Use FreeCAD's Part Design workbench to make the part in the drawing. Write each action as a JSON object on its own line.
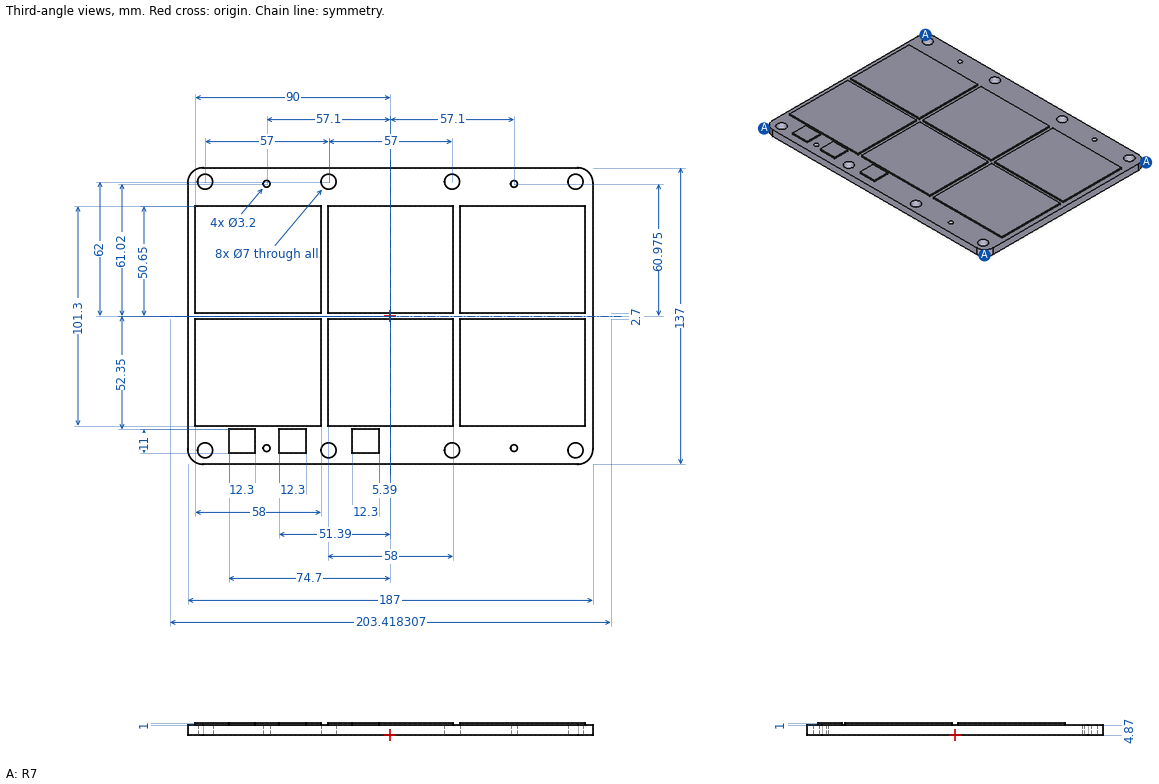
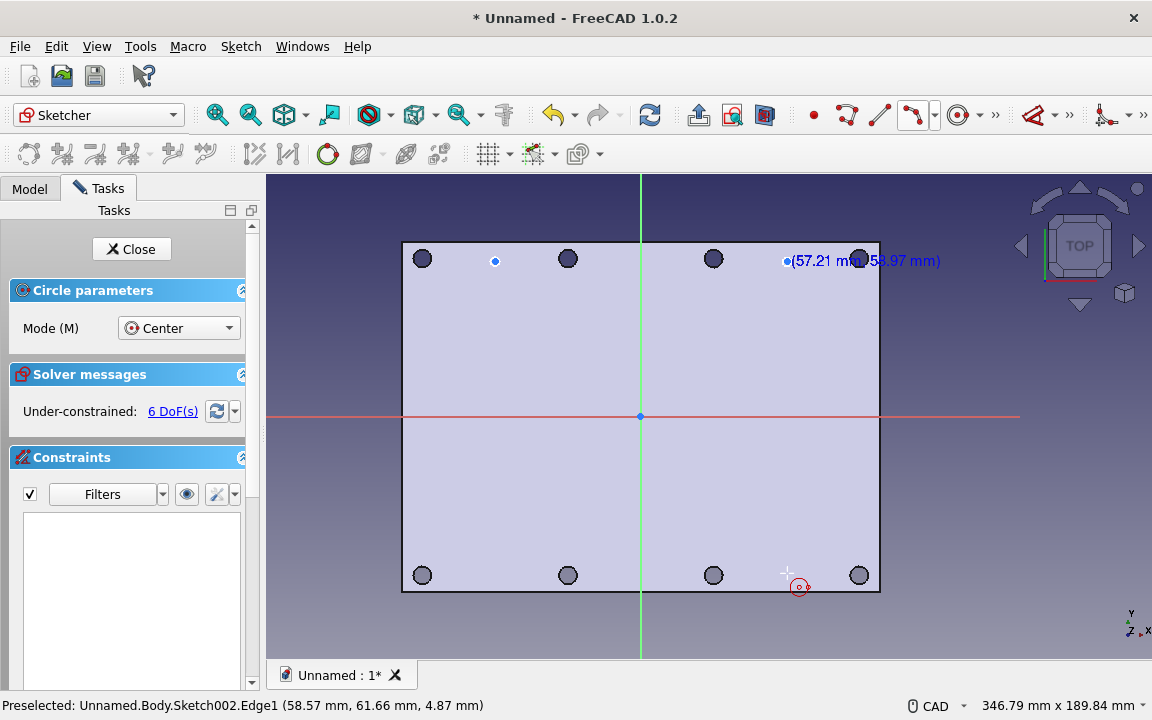
{"action": "left_click", "coordinate": [787, 573]}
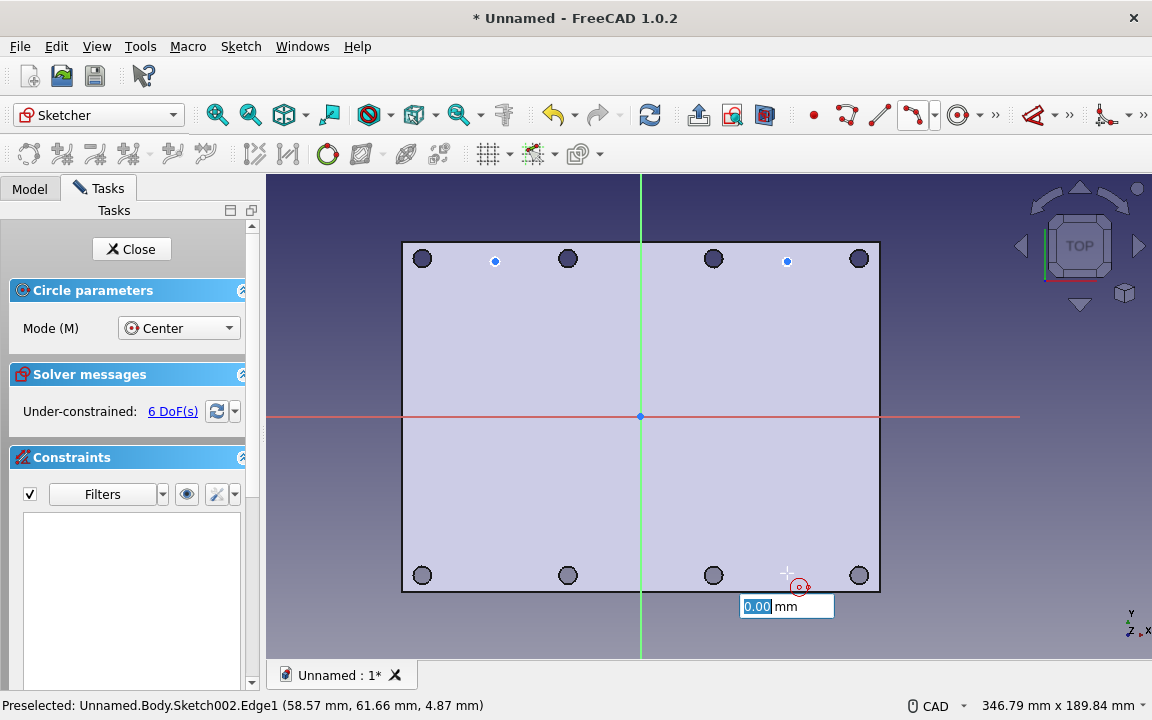
{"action": "scroll", "coordinate": [790, 570], "scroll_direction": "up", "scroll_amount": 7}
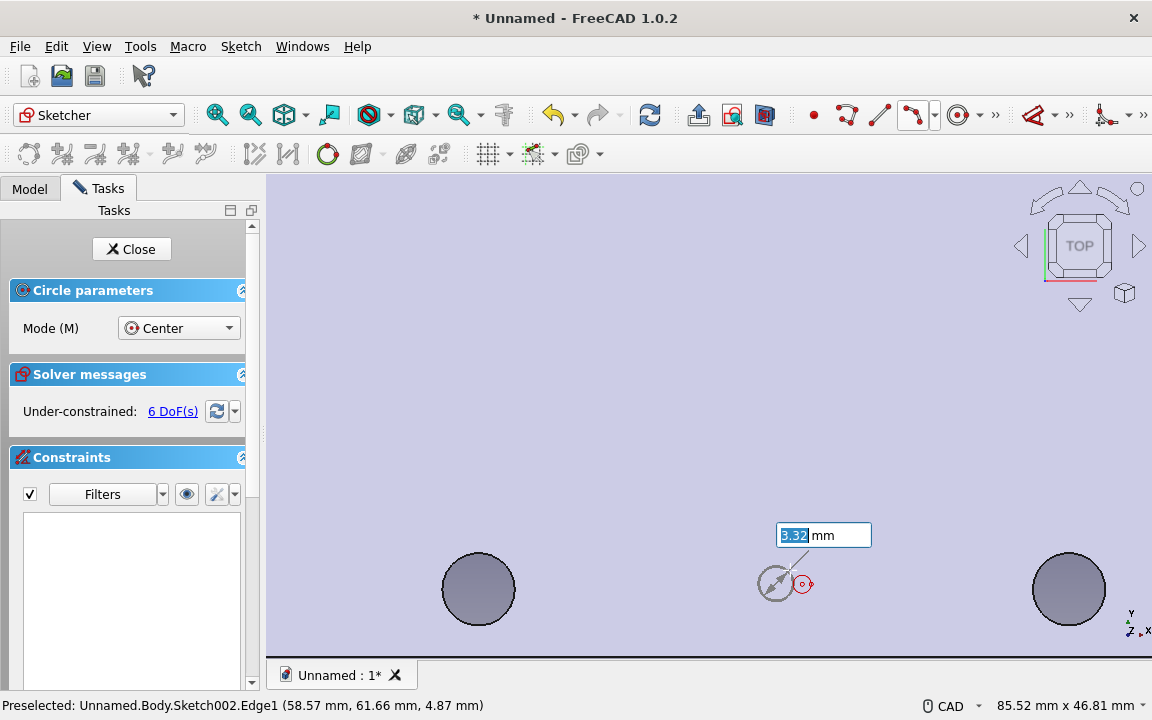
{"action": "left_click", "coordinate": [787, 567]}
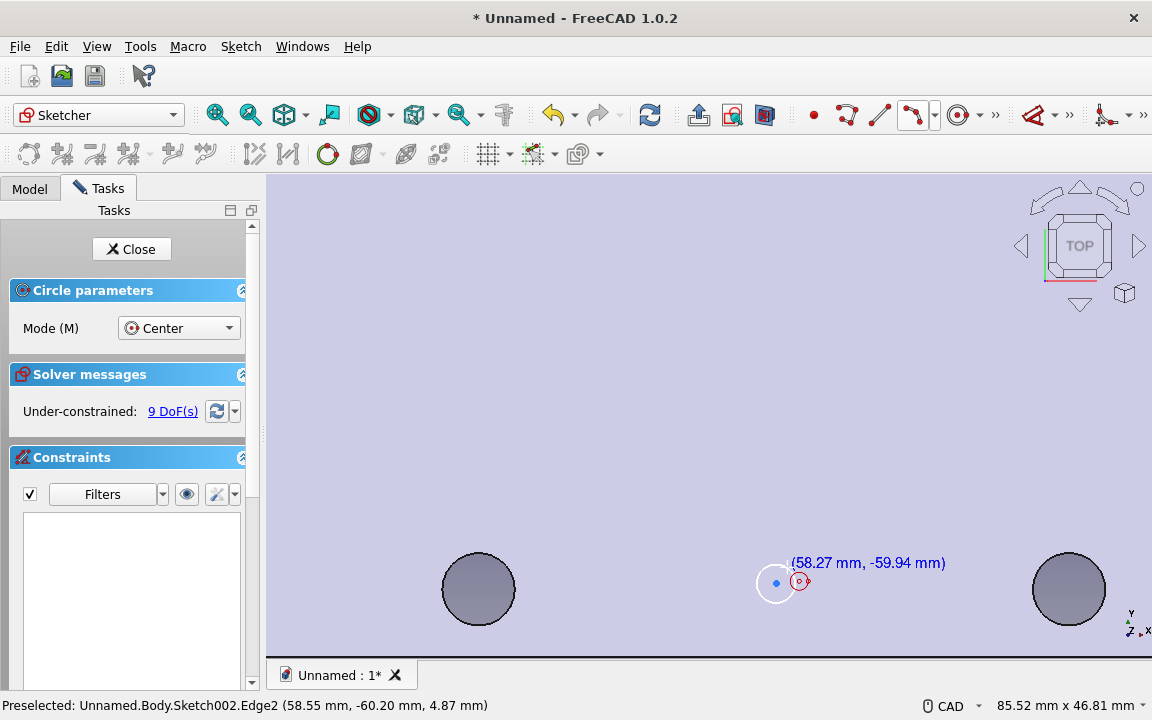
{"action": "scroll", "coordinate": [790, 570], "scroll_direction": "down", "scroll_amount": 7}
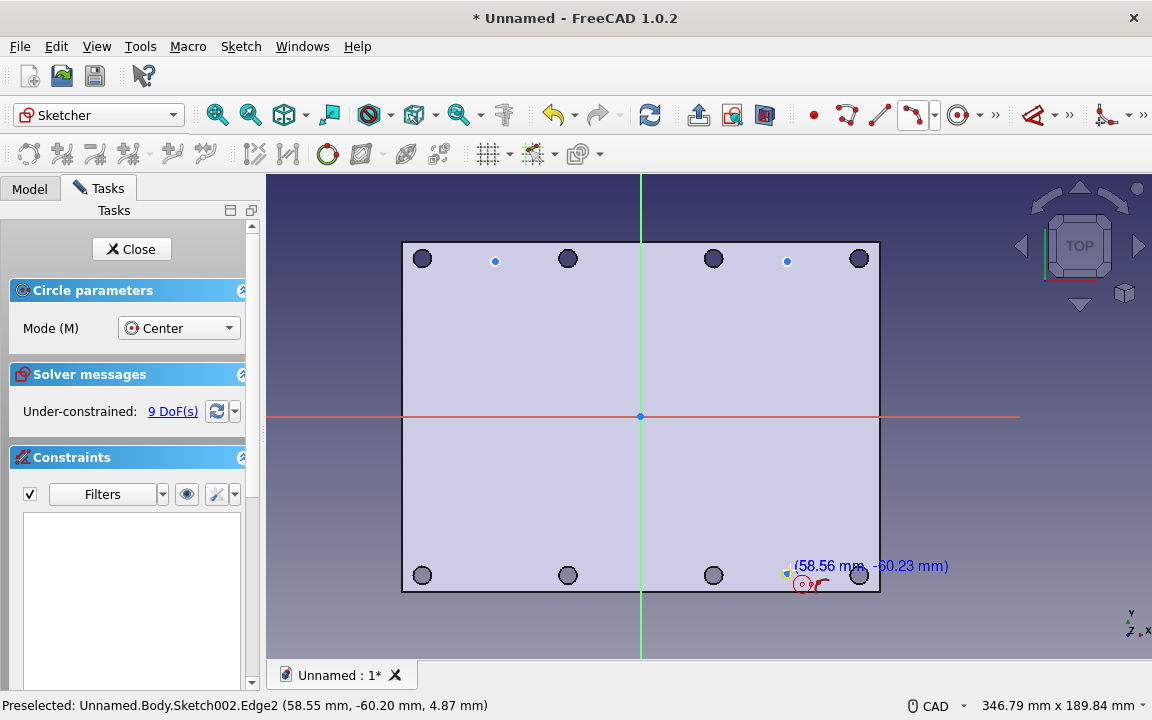
{"action": "scroll", "coordinate": [495, 573], "scroll_direction": "up", "scroll_amount": 9}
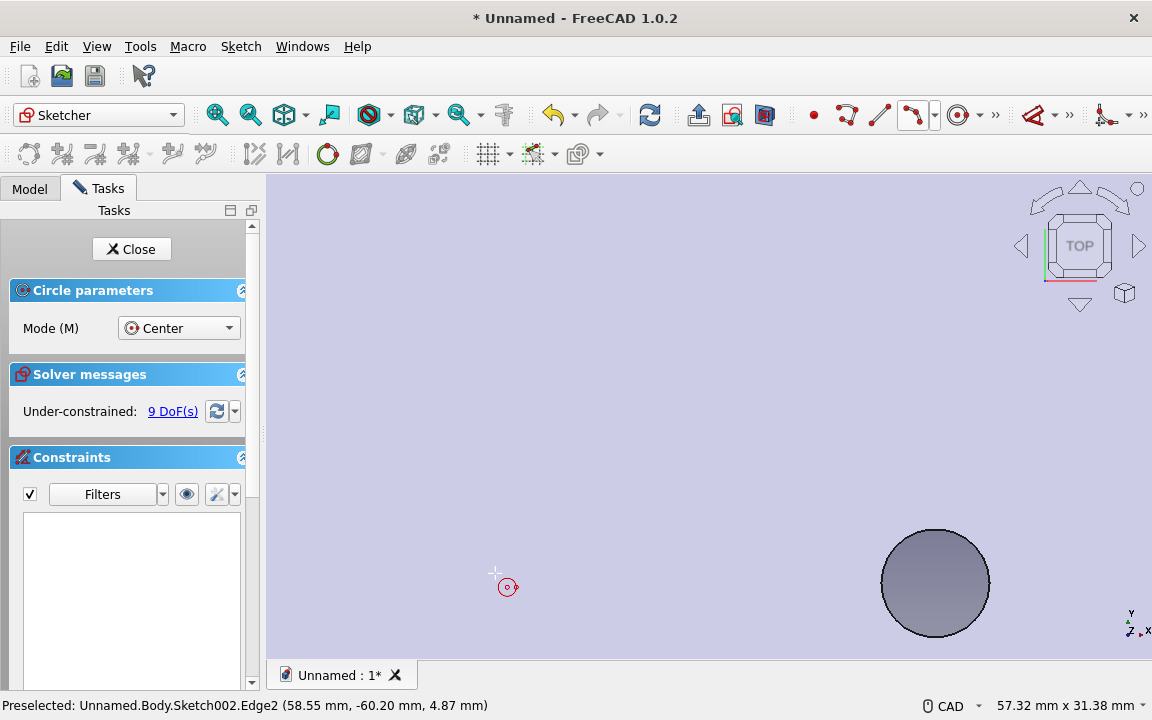
{"action": "scroll", "coordinate": [495, 573], "scroll_direction": "down", "scroll_amount": 9}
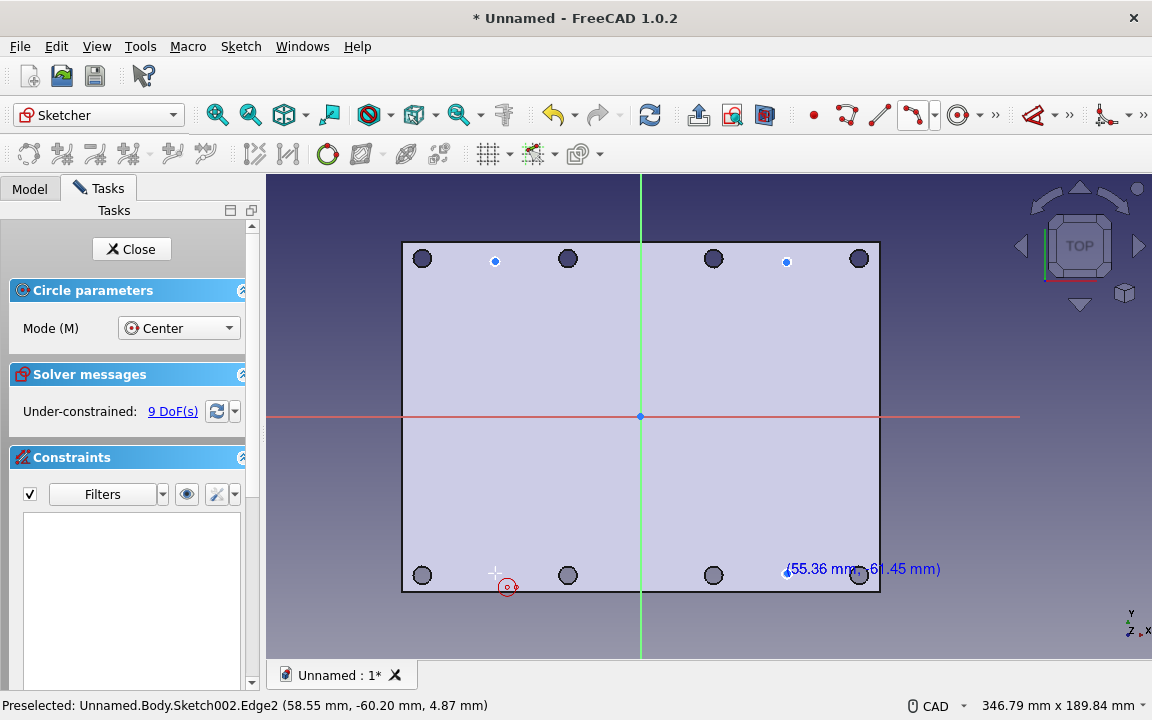
{"action": "left_click", "coordinate": [495, 573]}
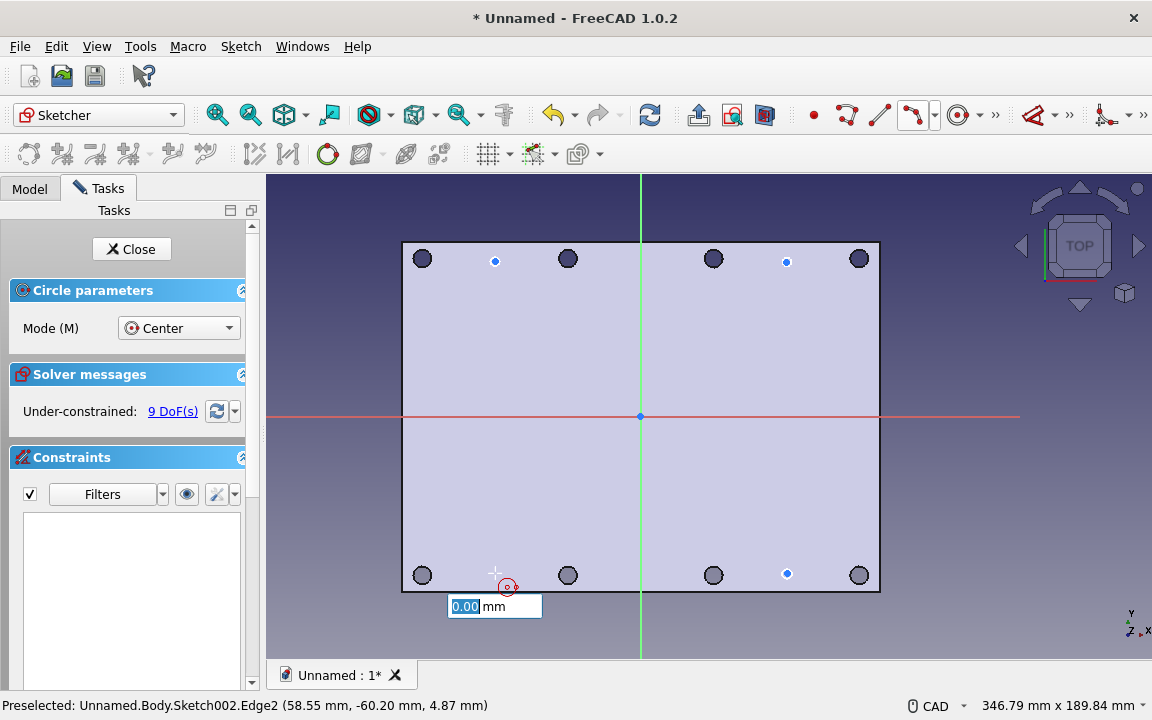
{"action": "scroll", "coordinate": [498, 570], "scroll_direction": "up", "scroll_amount": 7}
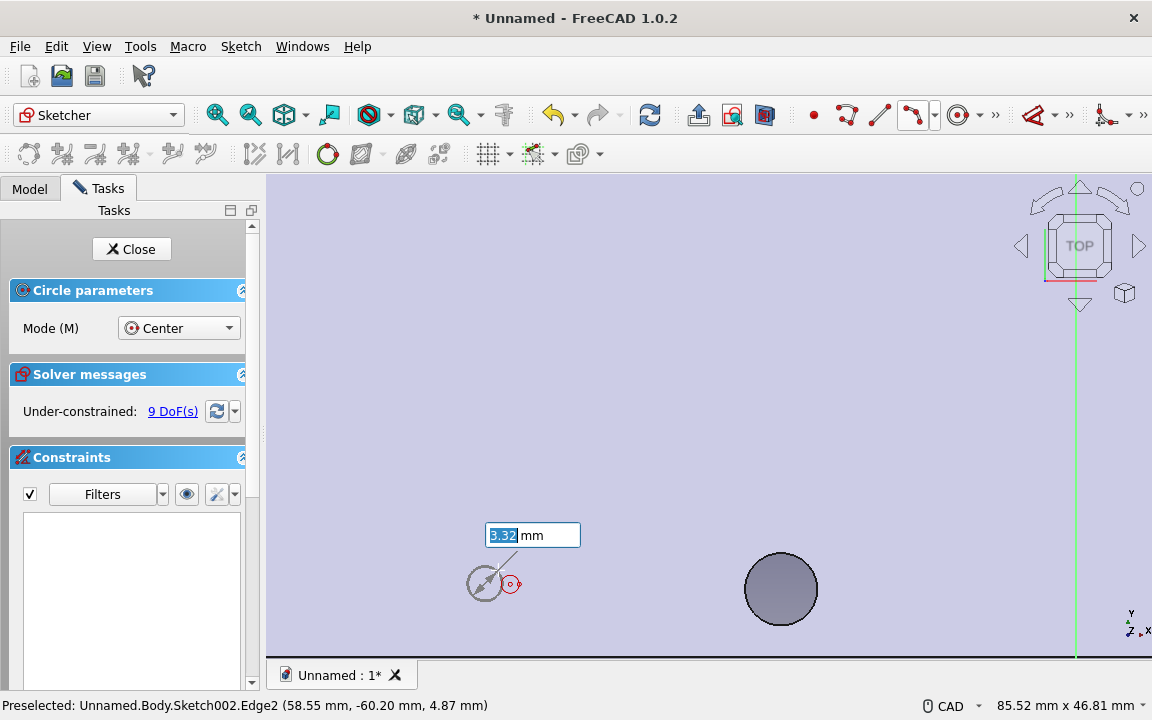
{"action": "left_click", "coordinate": [497, 567]}
{"action": "key", "text": "Escape"}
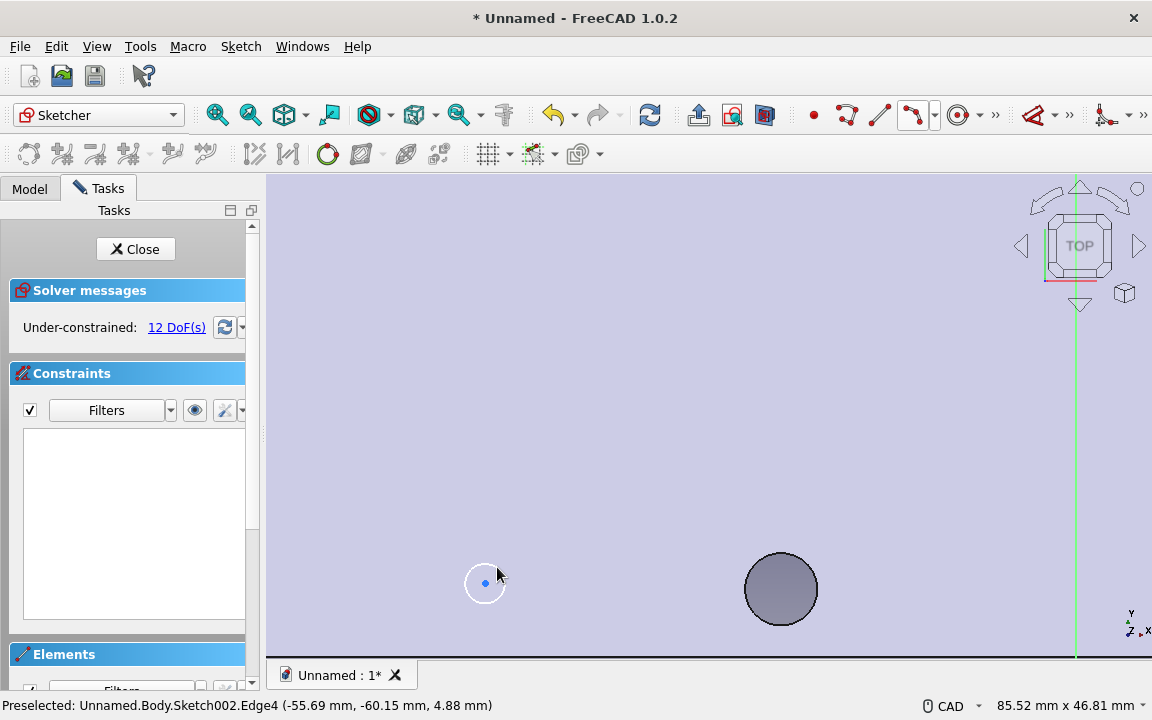
{"action": "scroll", "coordinate": [498, 570], "scroll_direction": "down", "scroll_amount": 7}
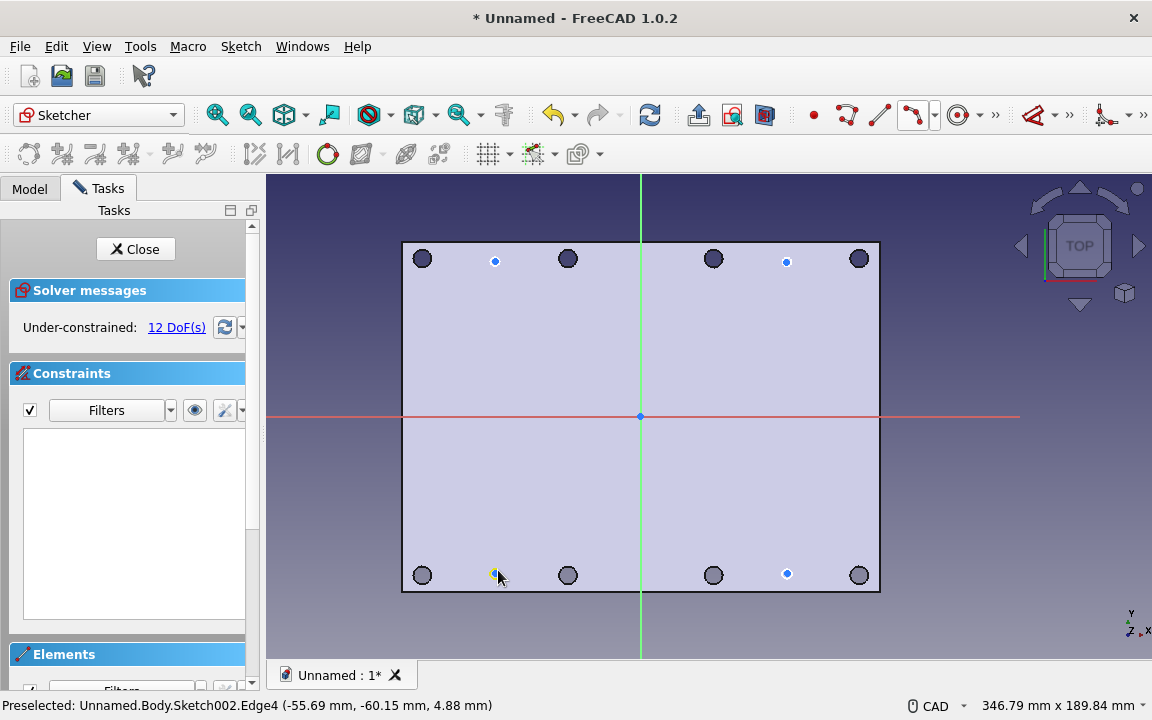
{"action": "scroll", "coordinate": [498, 259], "scroll_direction": "up", "scroll_amount": 6}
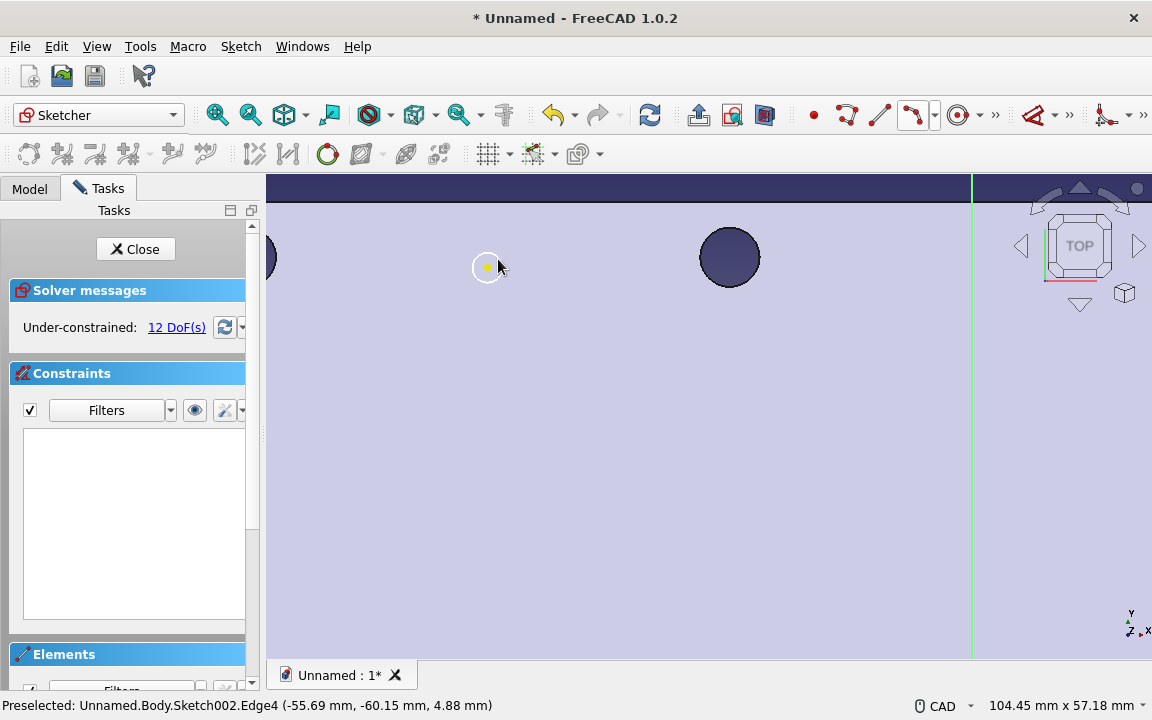
{"action": "left_click", "coordinate": [498, 257]}